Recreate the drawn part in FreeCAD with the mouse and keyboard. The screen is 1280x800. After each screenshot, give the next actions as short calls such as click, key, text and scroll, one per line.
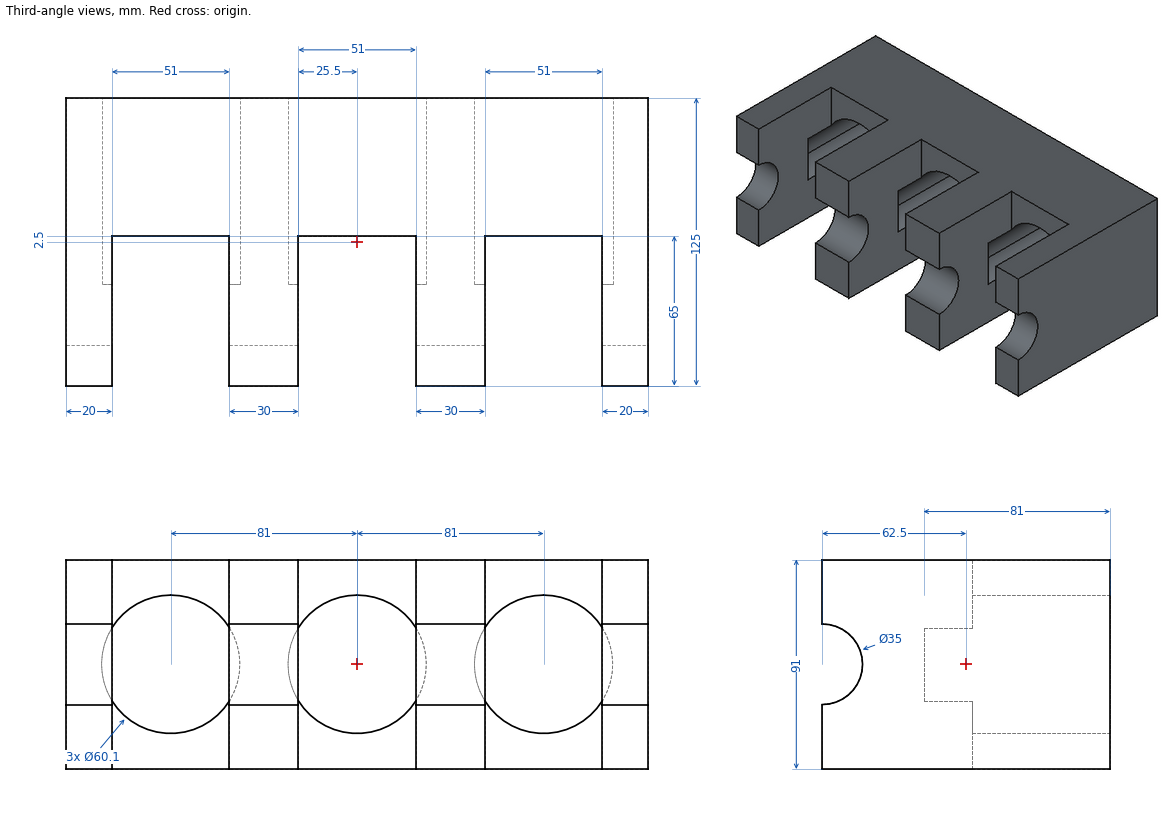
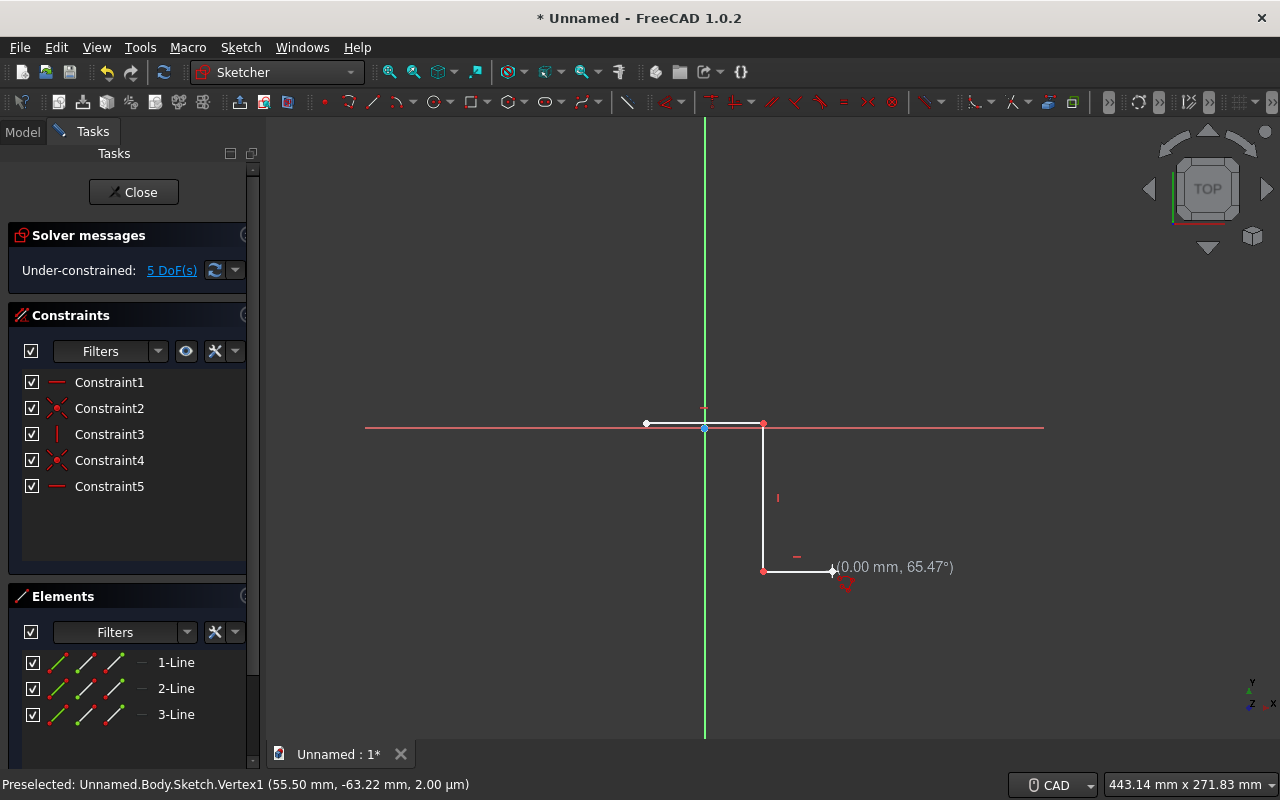
scroll(832, 423, up, 6)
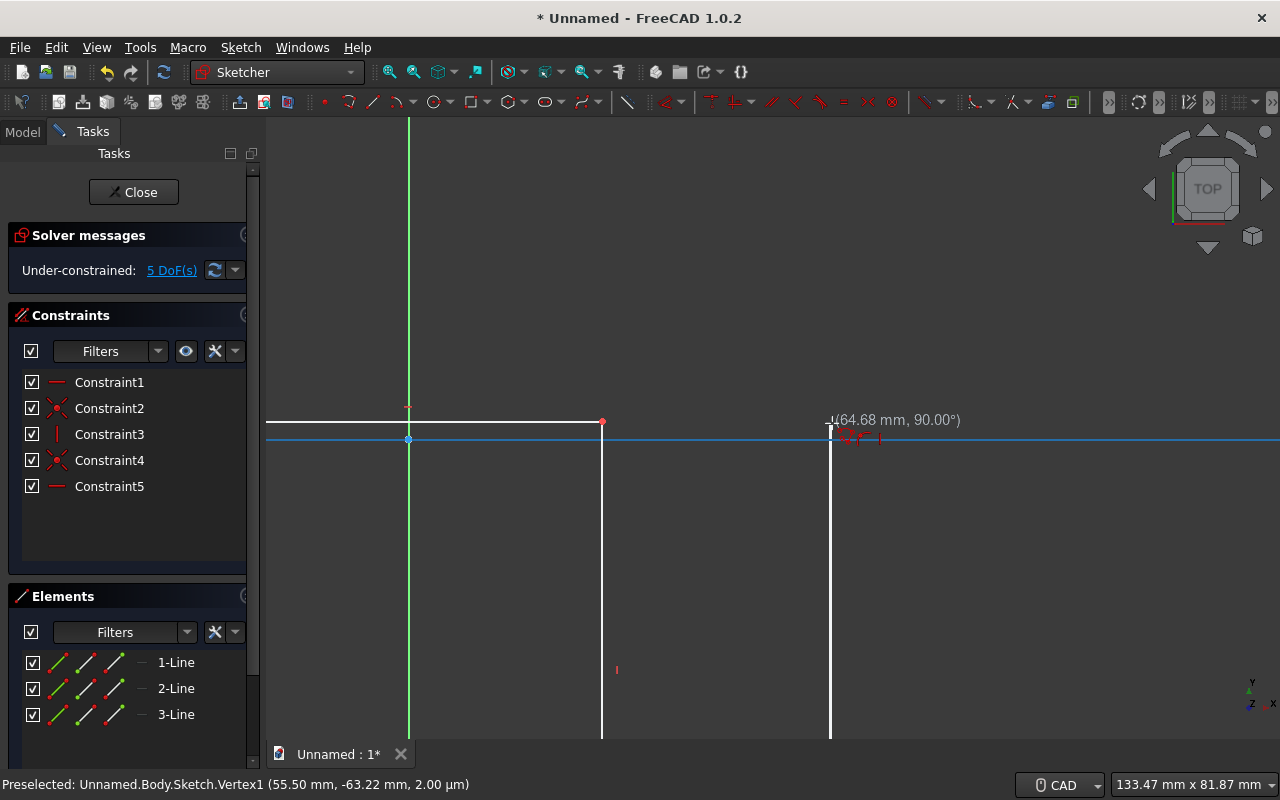
click(831, 421)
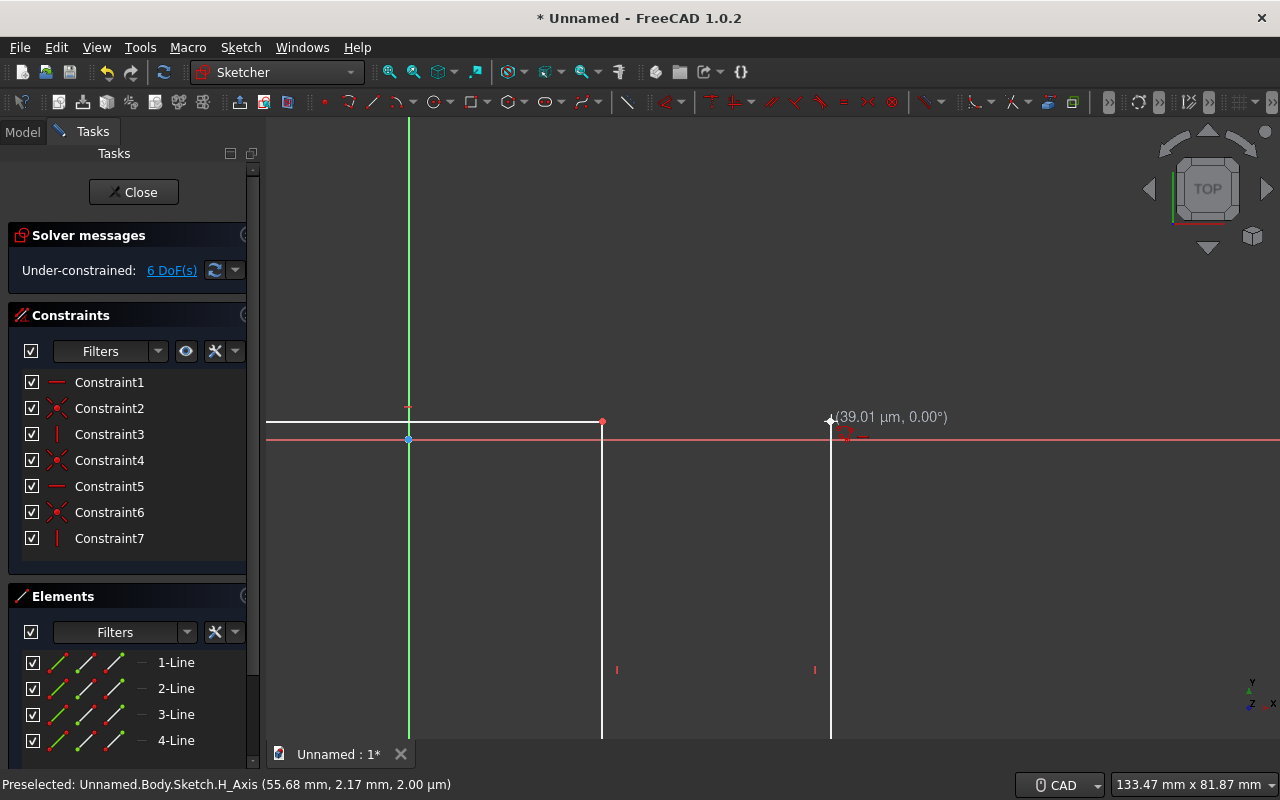
scroll(832, 423, down, 6)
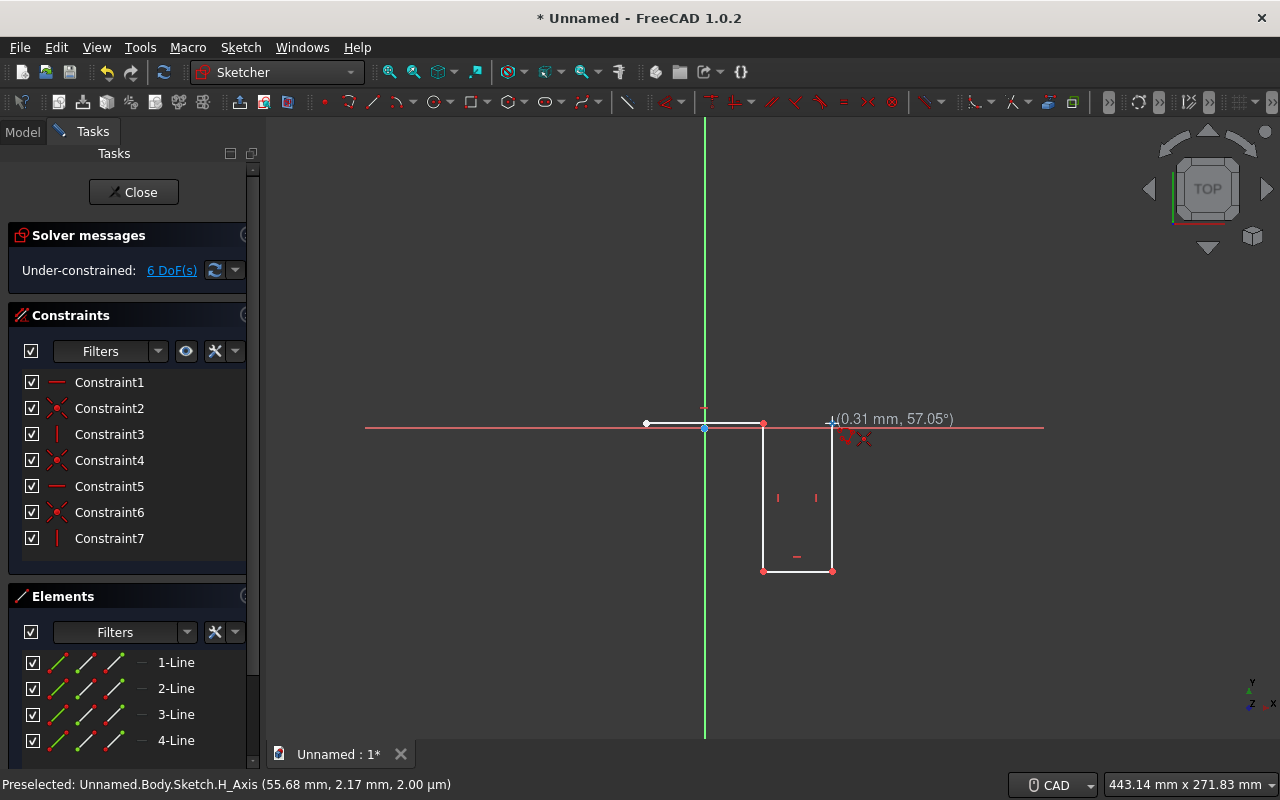
scroll(949, 423, up, 6)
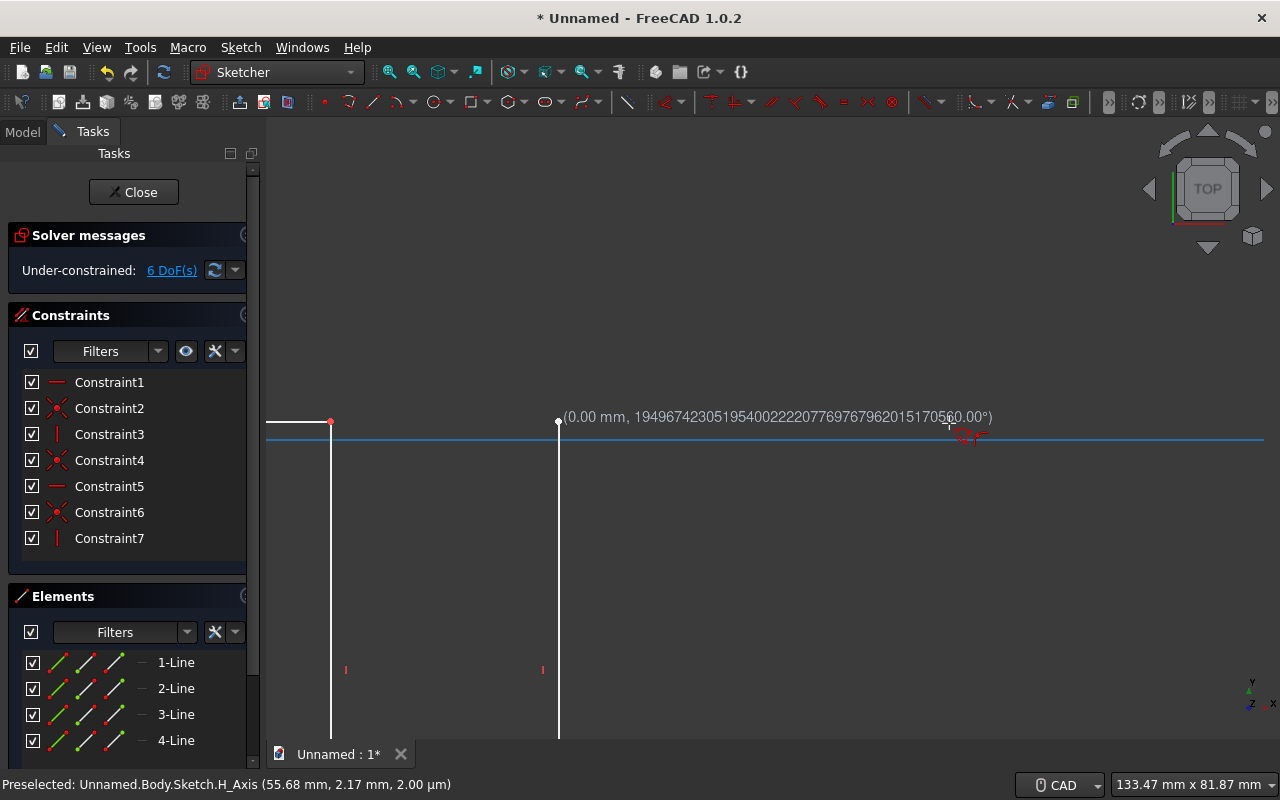
click(946, 421)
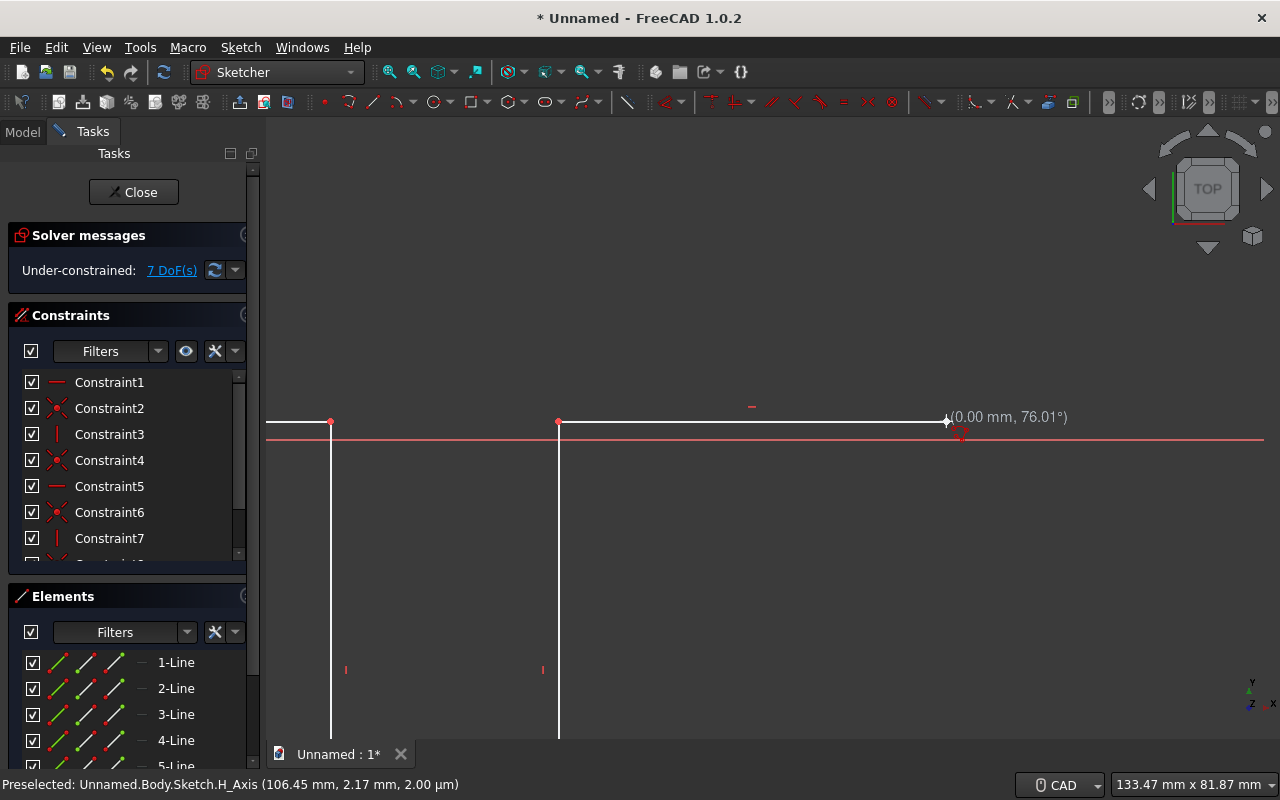
scroll(949, 423, down, 6)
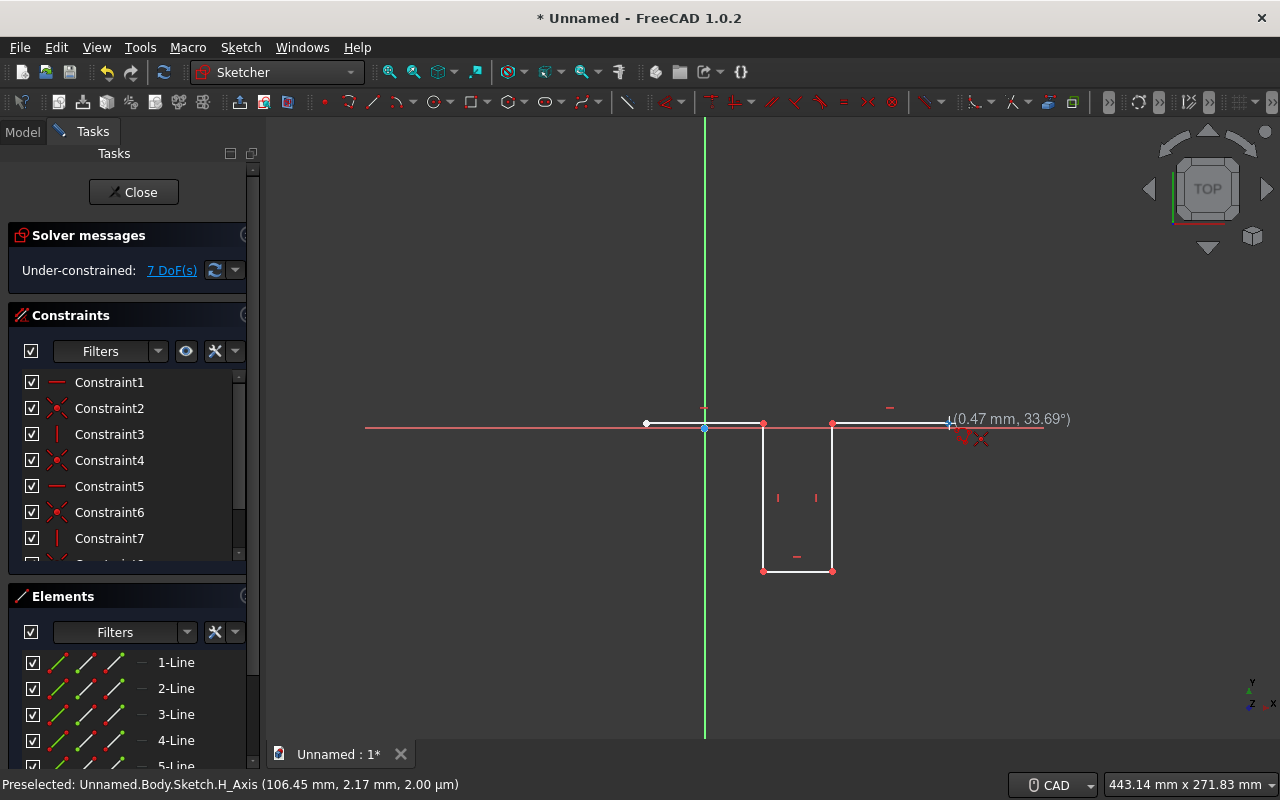
click(949, 571)
click(994, 571)
click(994, 285)
click(416, 285)
click(416, 571)
click(461, 571)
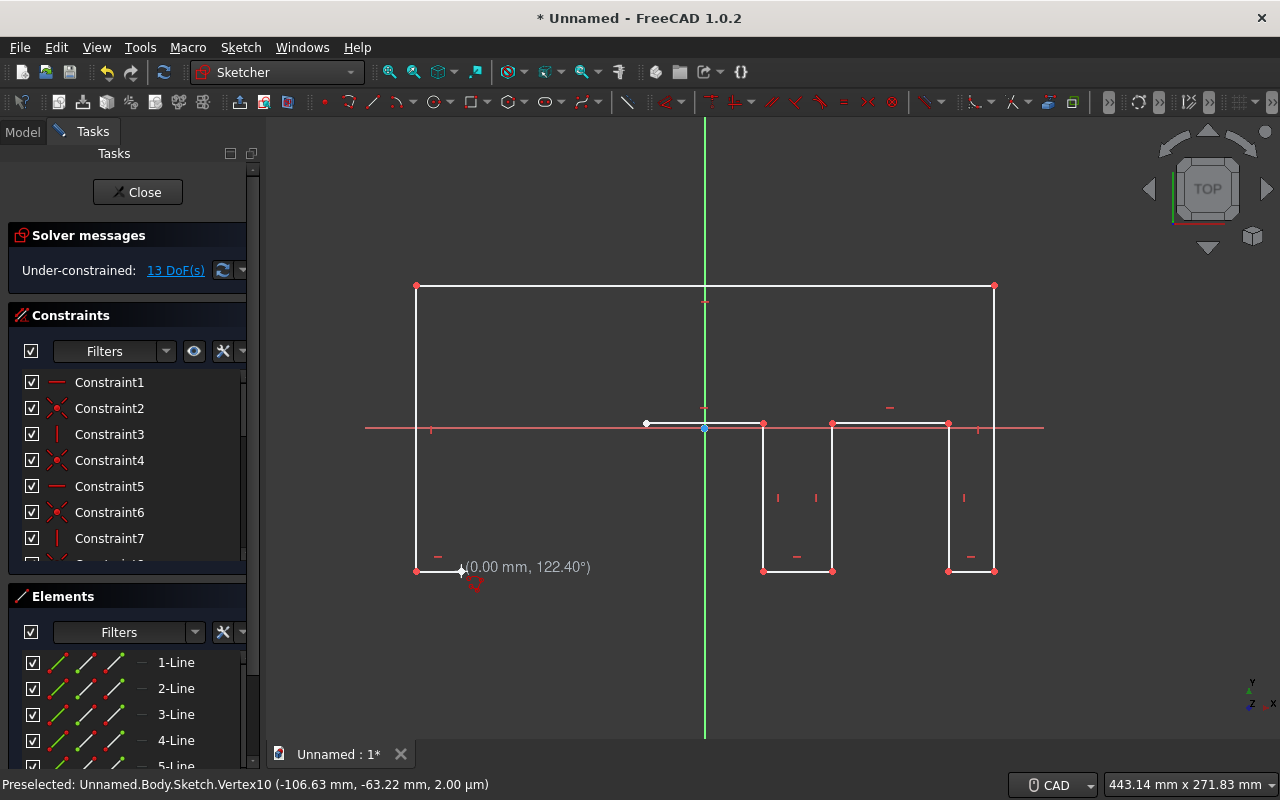
scroll(461, 423, up, 6)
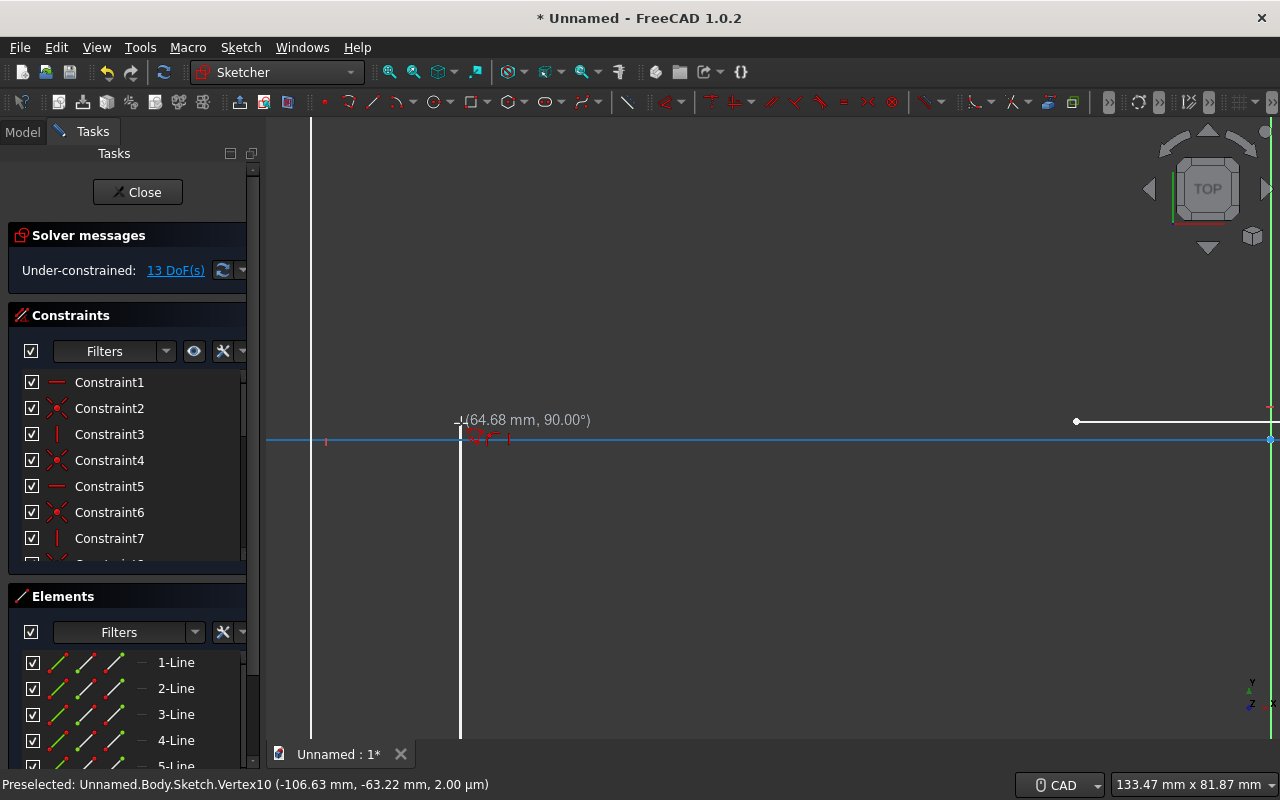
click(461, 421)
click(849, 421)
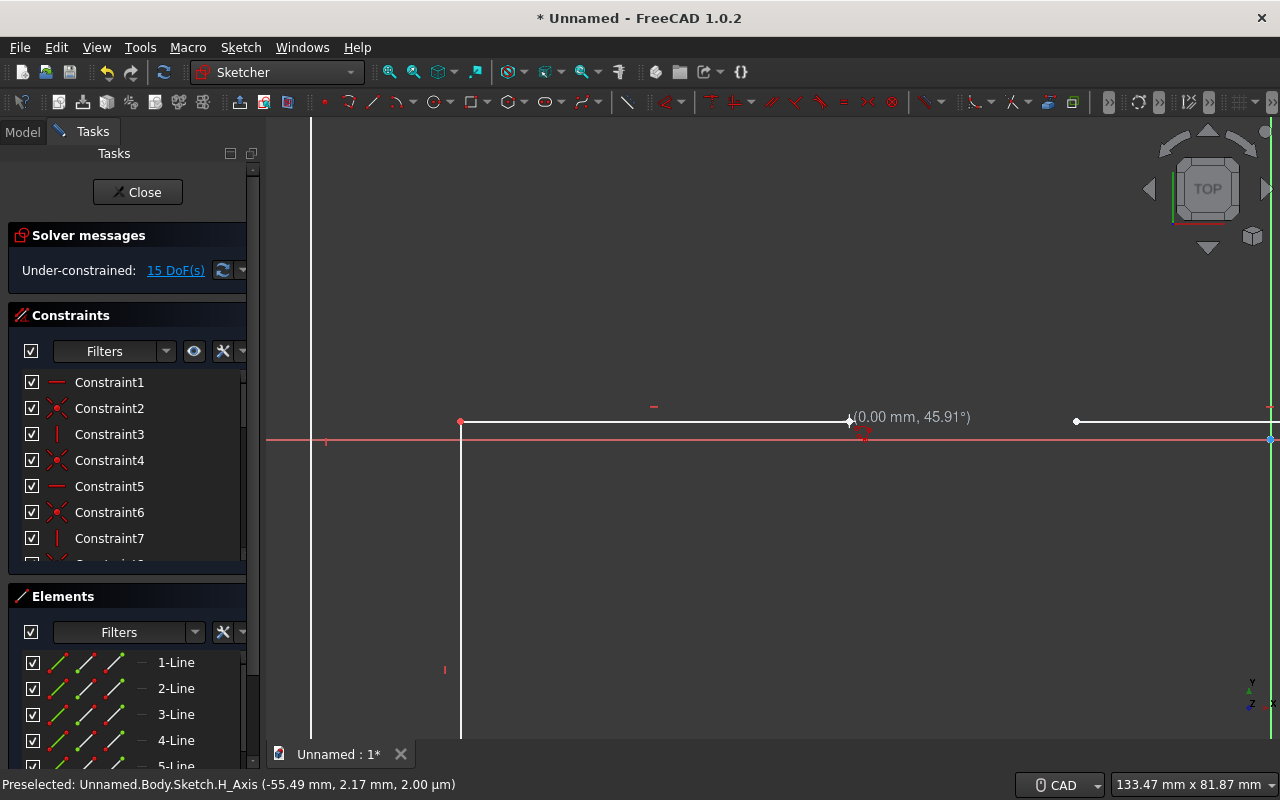
scroll(461, 423, down, 6)